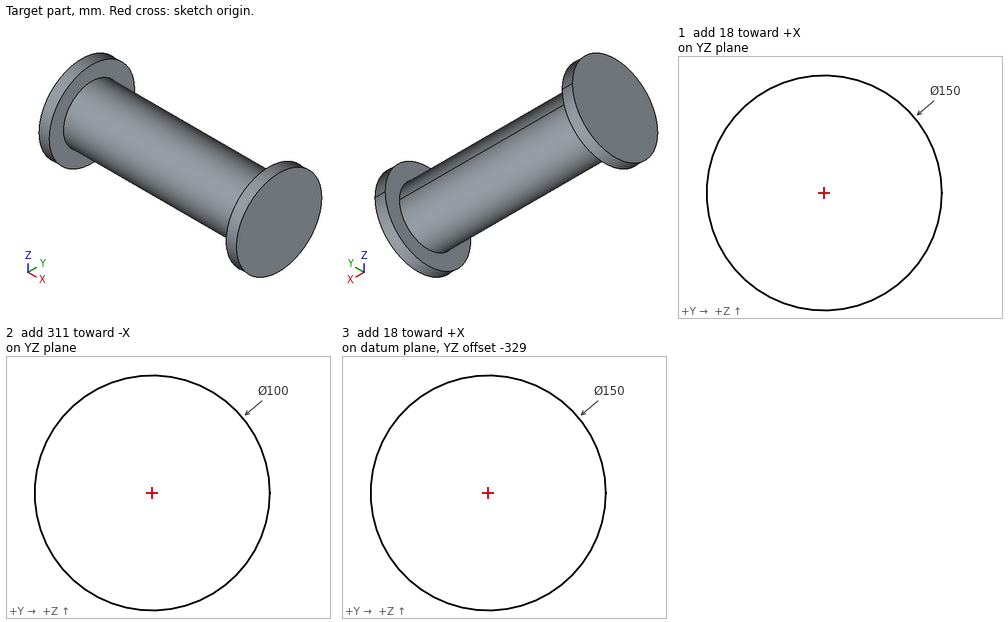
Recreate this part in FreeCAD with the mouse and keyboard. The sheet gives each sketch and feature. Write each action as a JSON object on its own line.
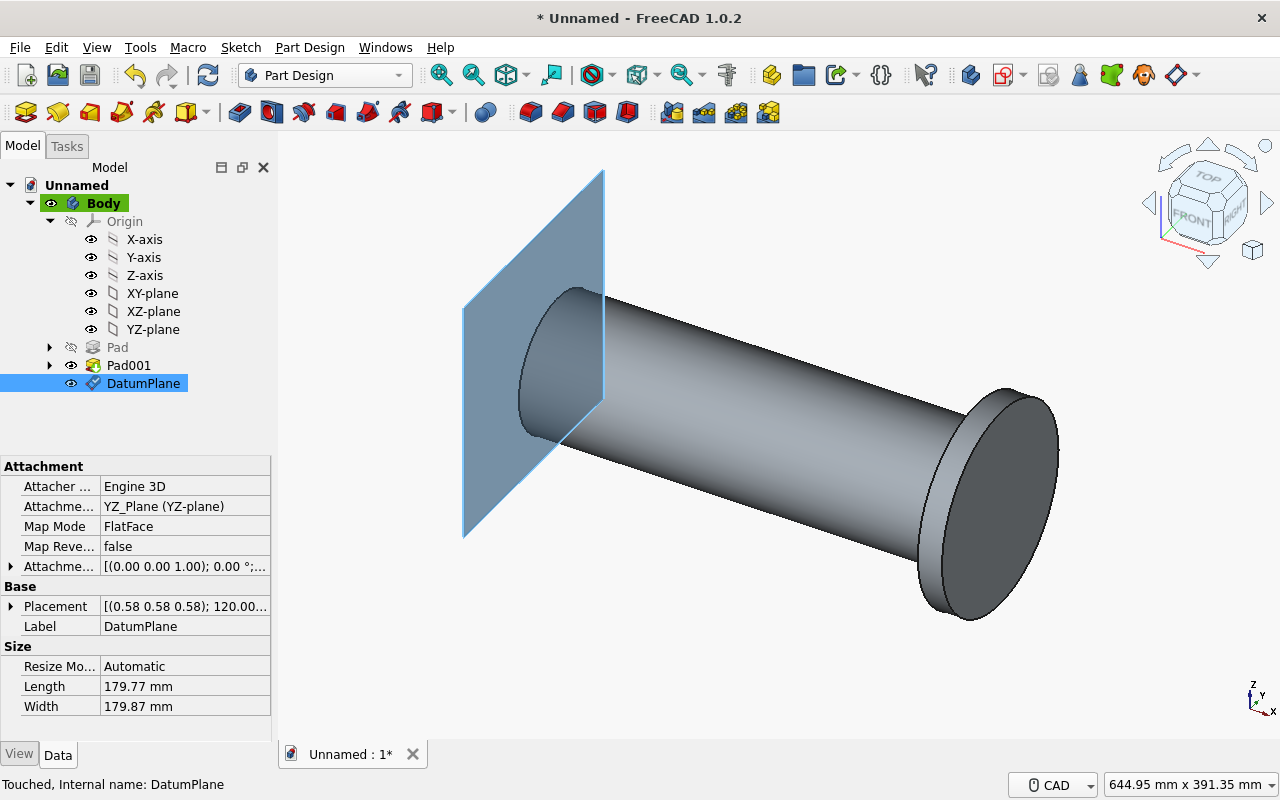
{"action": "left_click", "coordinate": [1004, 76]}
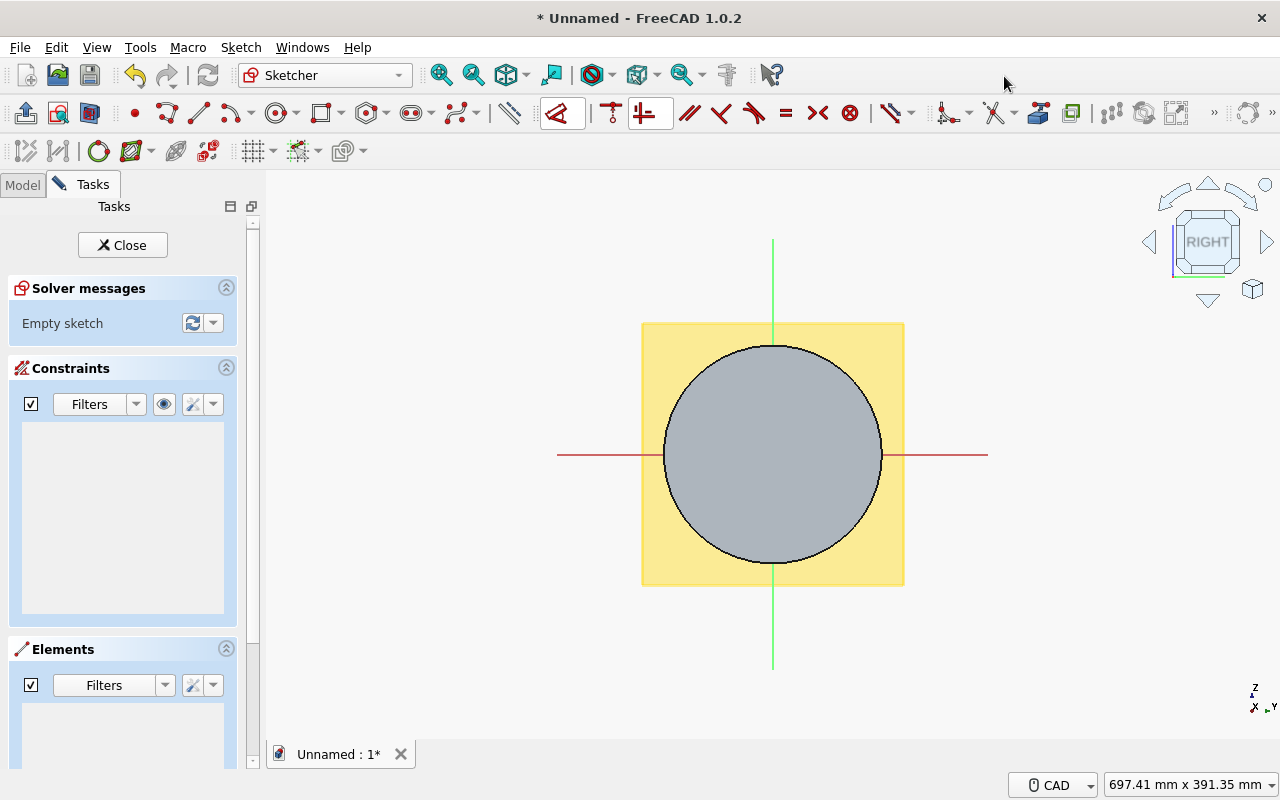
{"action": "key", "text": "q s"}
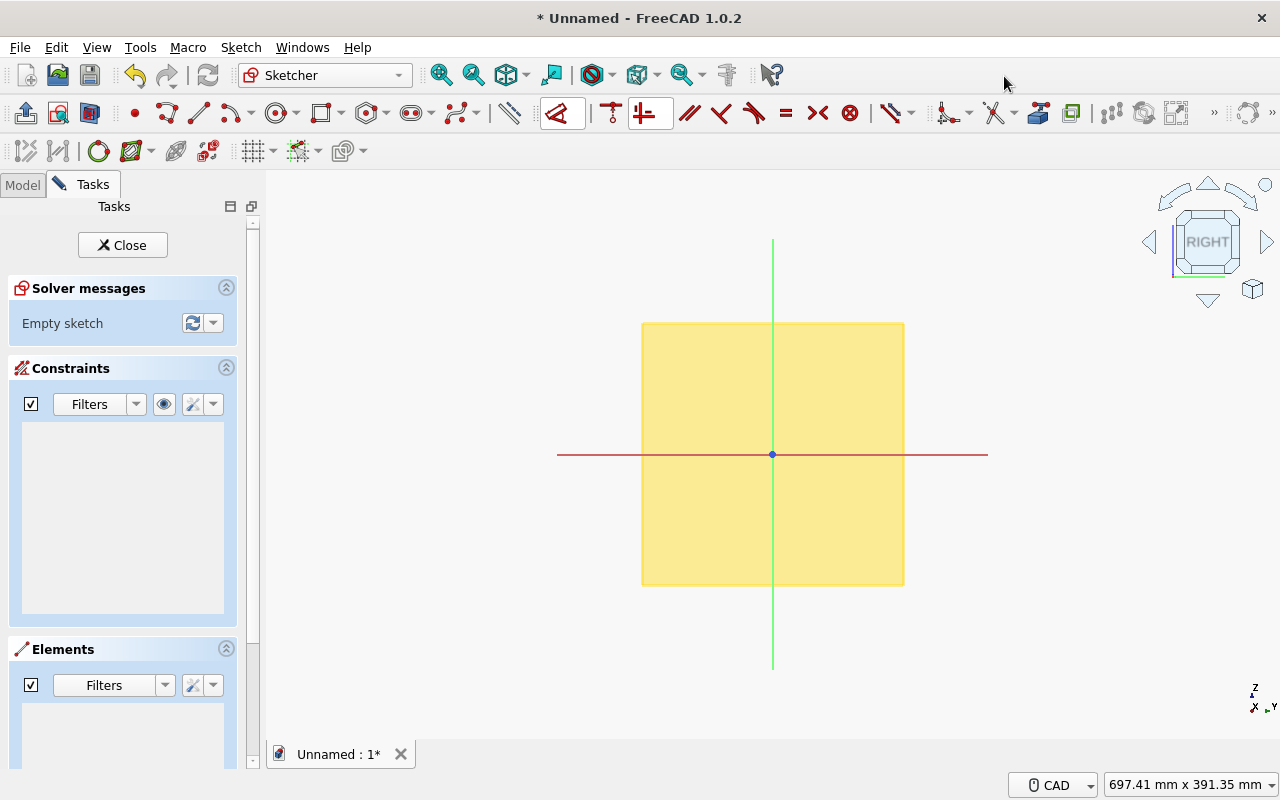
{"action": "scroll", "coordinate": [856, 454], "scroll_direction": "up", "scroll_amount": 3}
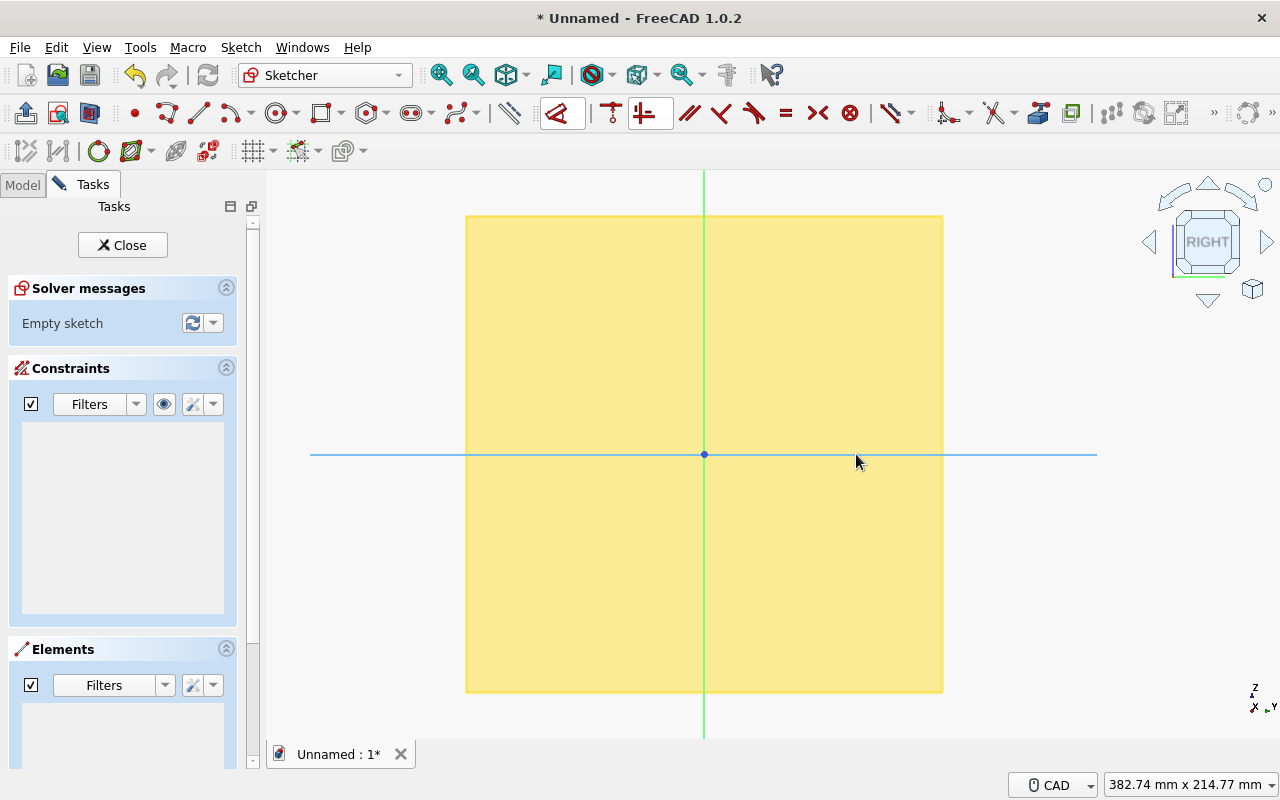
{"action": "key", "text": "g c"}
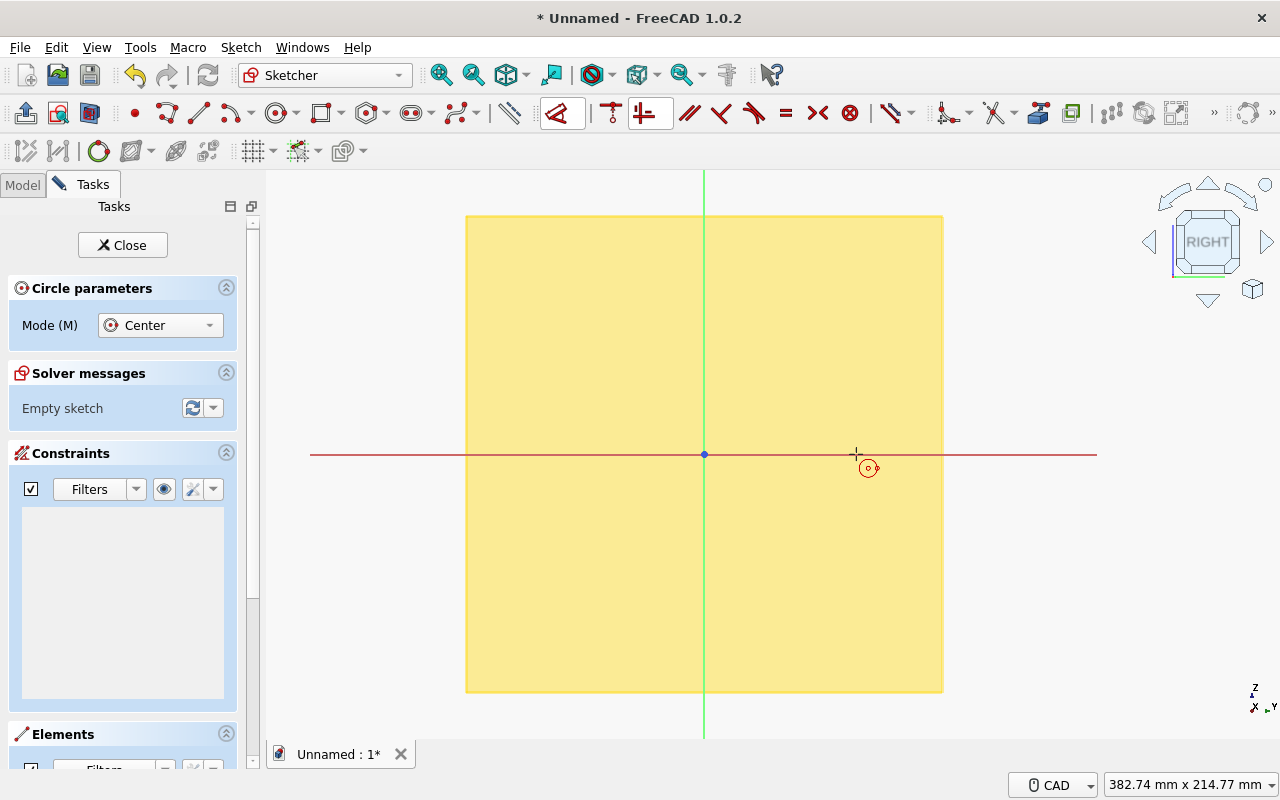
{"action": "left_click", "coordinate": [704, 454]}
{"action": "left_click", "coordinate": [845, 314]}
{"action": "key", "text": "Escape"}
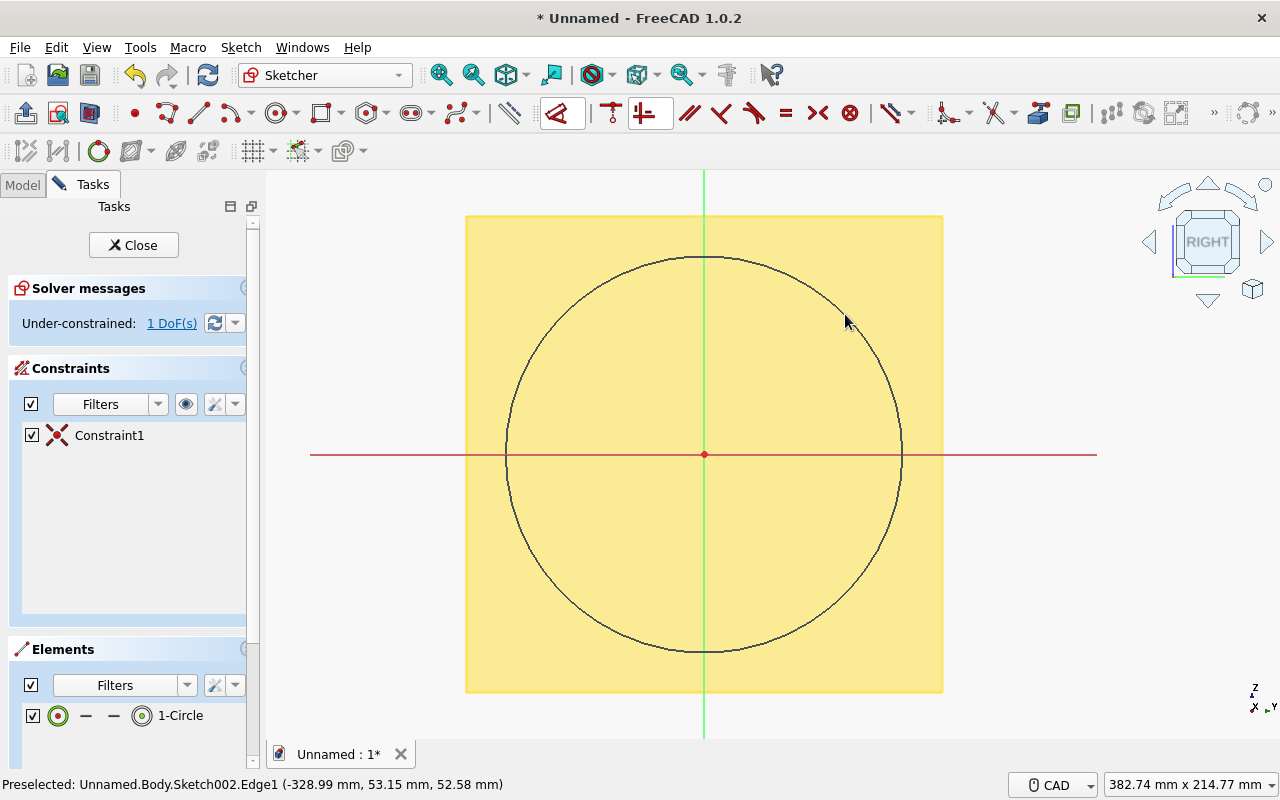
{"action": "left_click", "coordinate": [844, 314]}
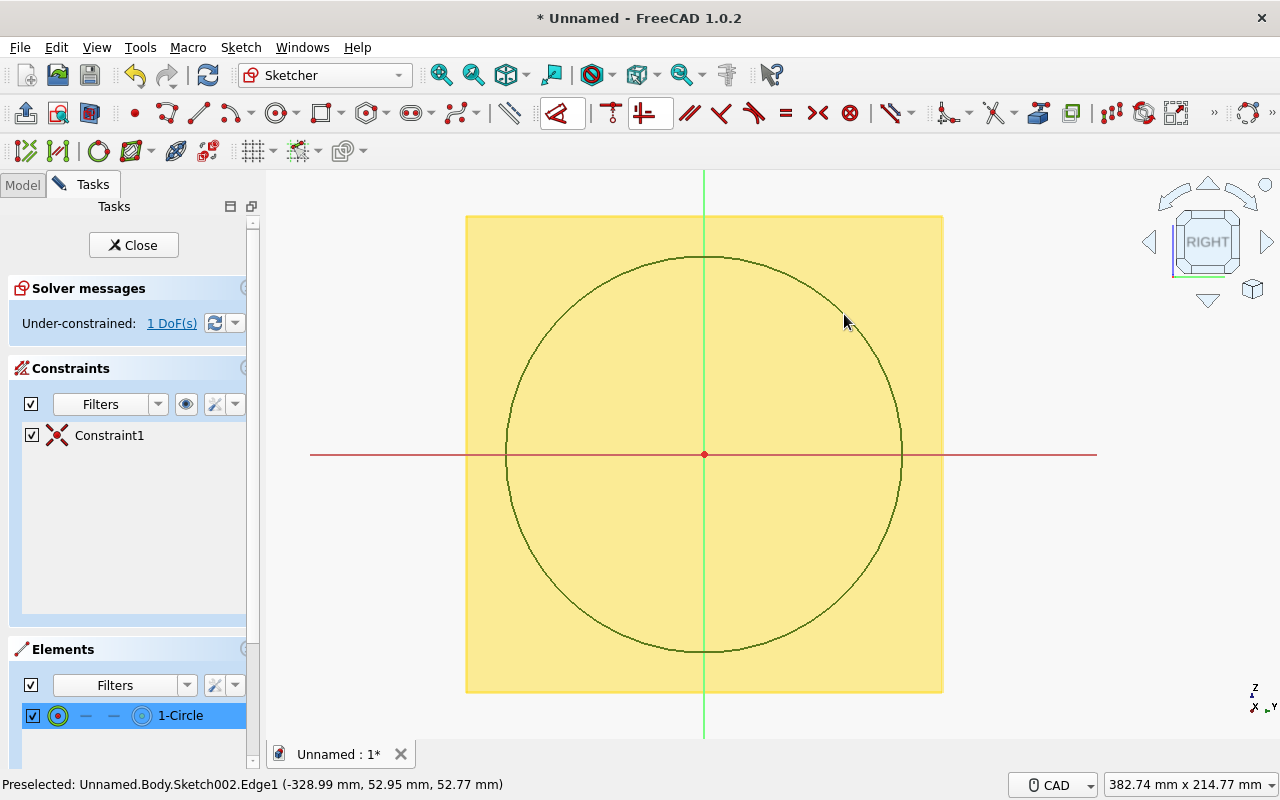
{"action": "key", "text": "k o"}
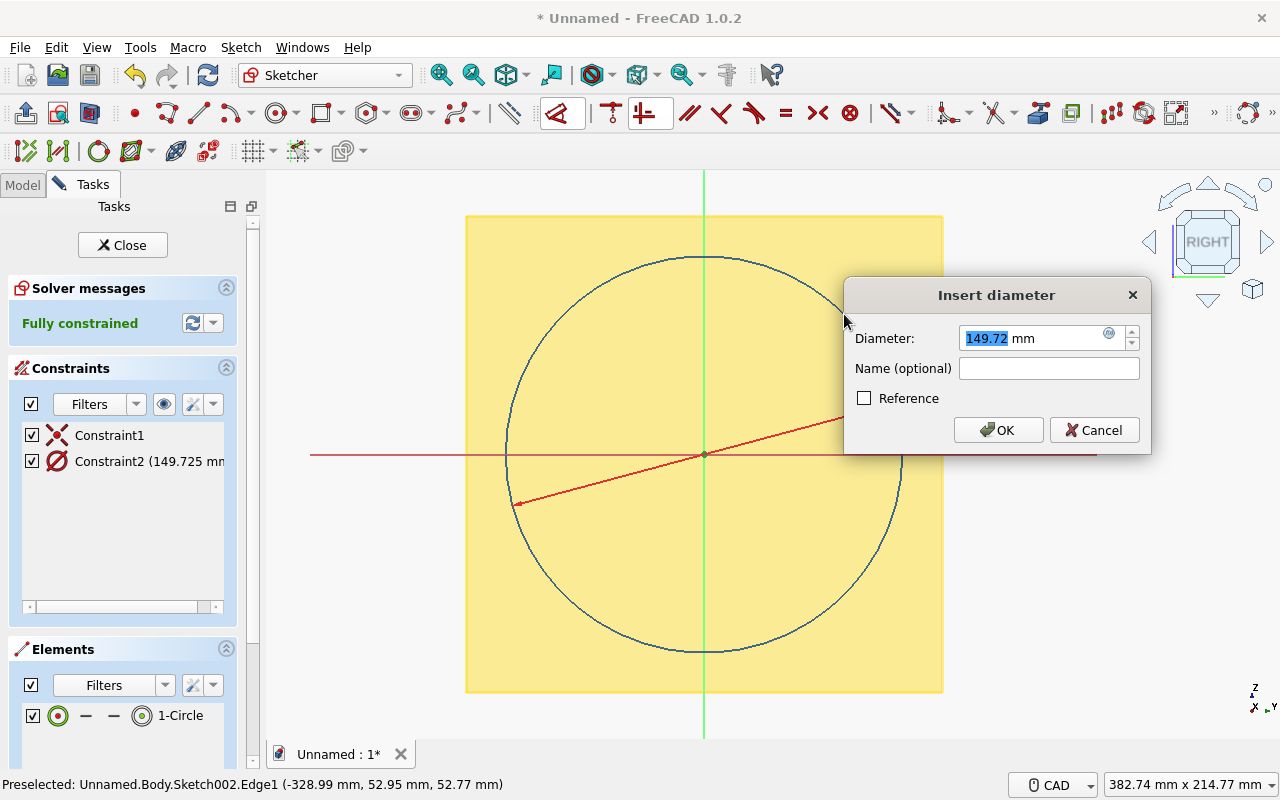
{"action": "type", "text": "150"}
{"action": "key", "text": "Return"}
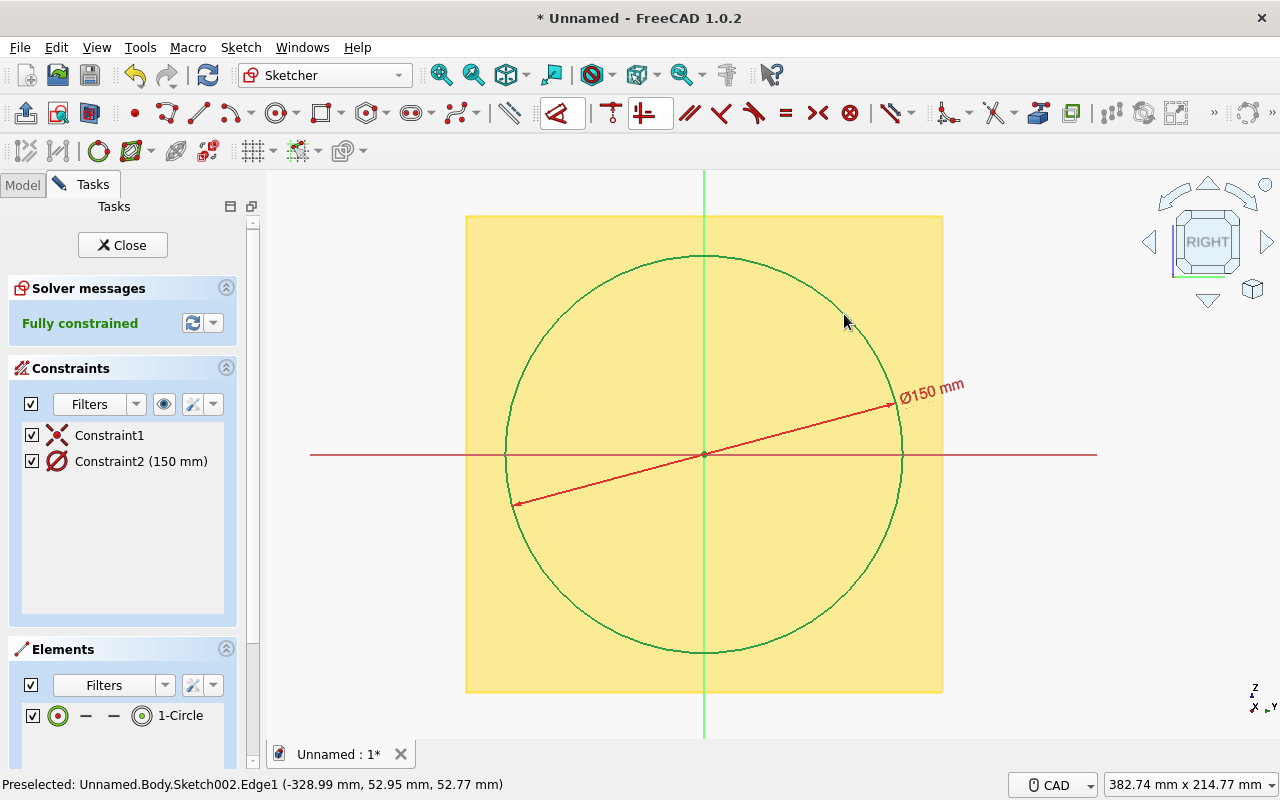
{"action": "left_click", "coordinate": [123, 245]}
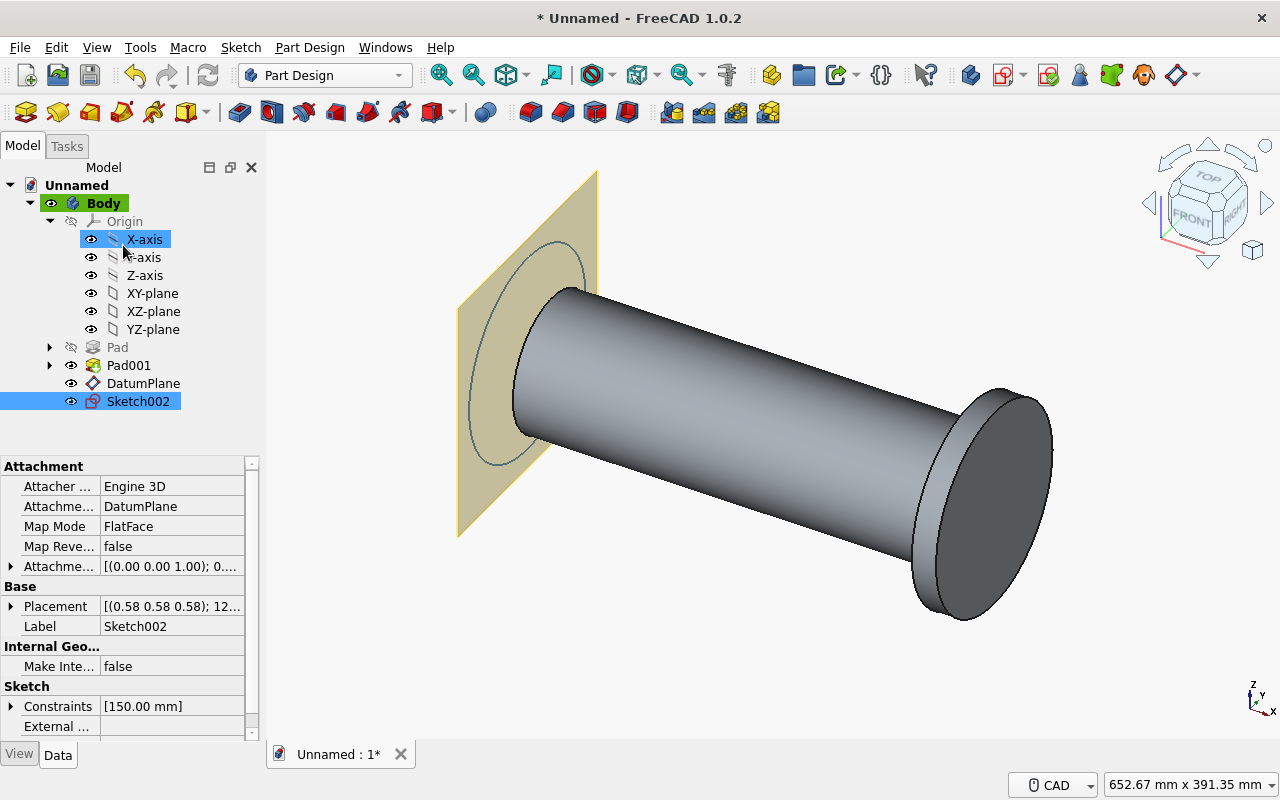
{"action": "left_click", "coordinate": [26, 112]}